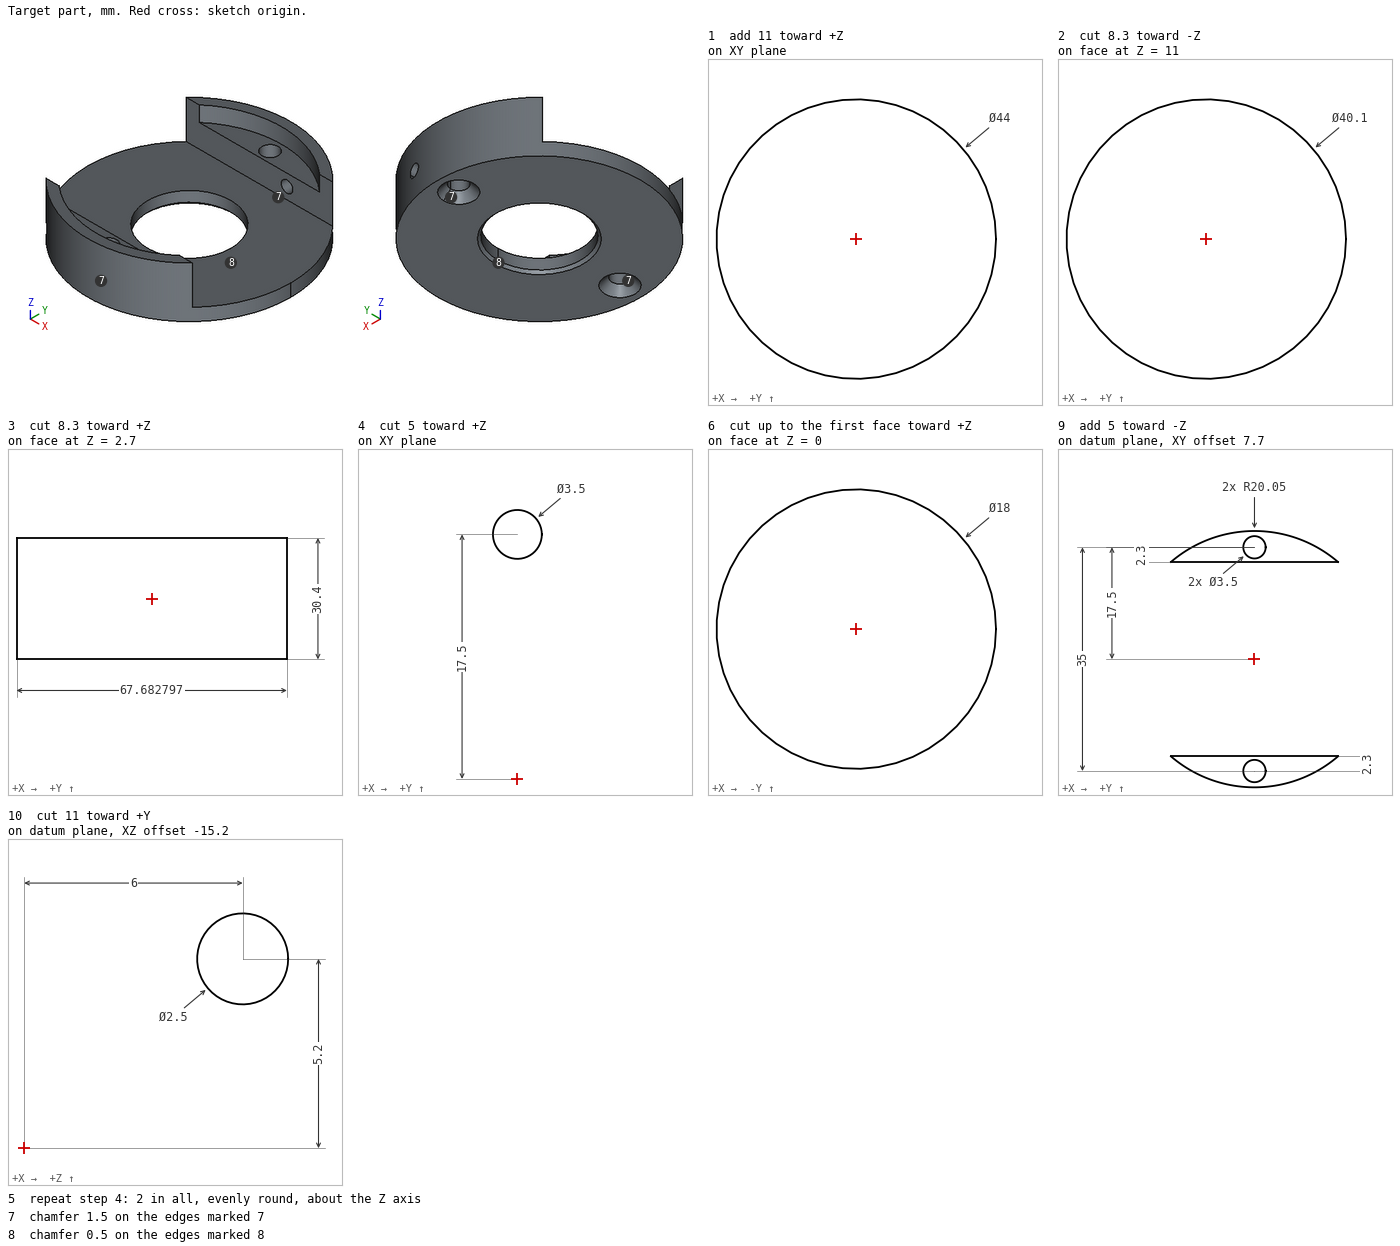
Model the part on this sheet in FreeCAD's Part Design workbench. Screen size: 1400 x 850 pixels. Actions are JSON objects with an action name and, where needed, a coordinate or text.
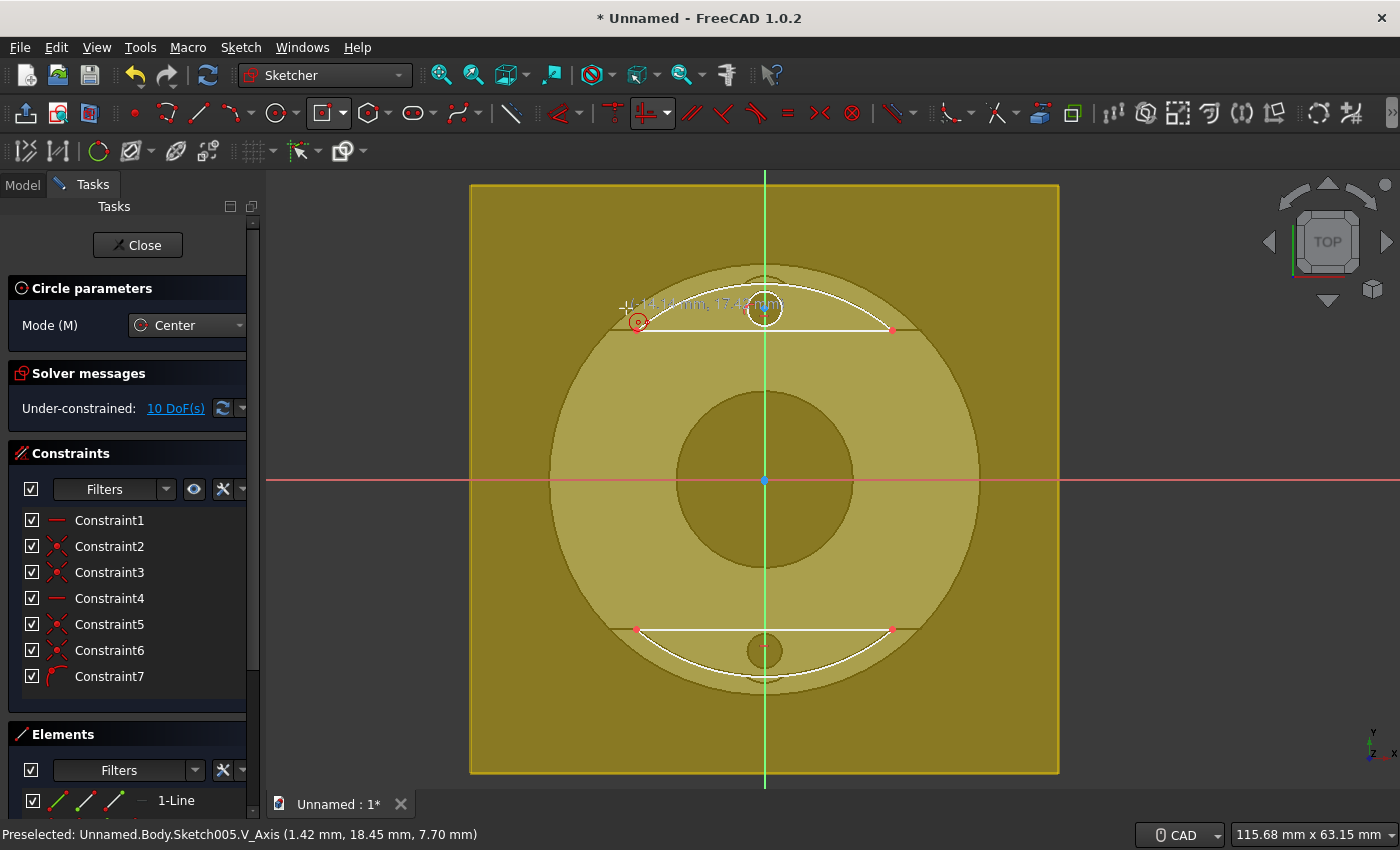
{"action": "scroll", "coordinate": [765, 651], "scroll_direction": "up", "scroll_amount": 2}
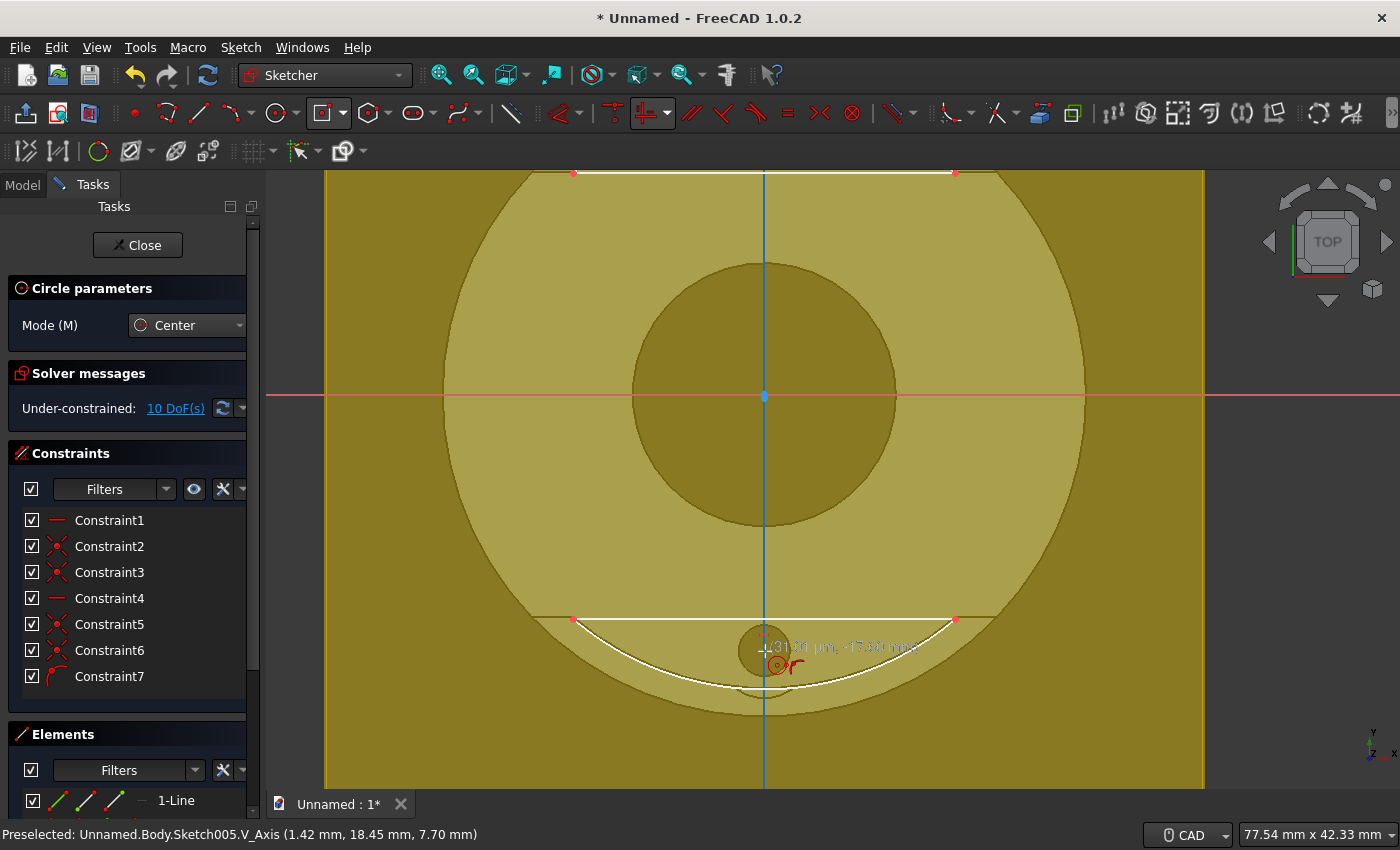
{"action": "left_click", "coordinate": [764, 651]}
{"action": "left_click", "coordinate": [782, 633]}
{"action": "key", "text": "Escape"}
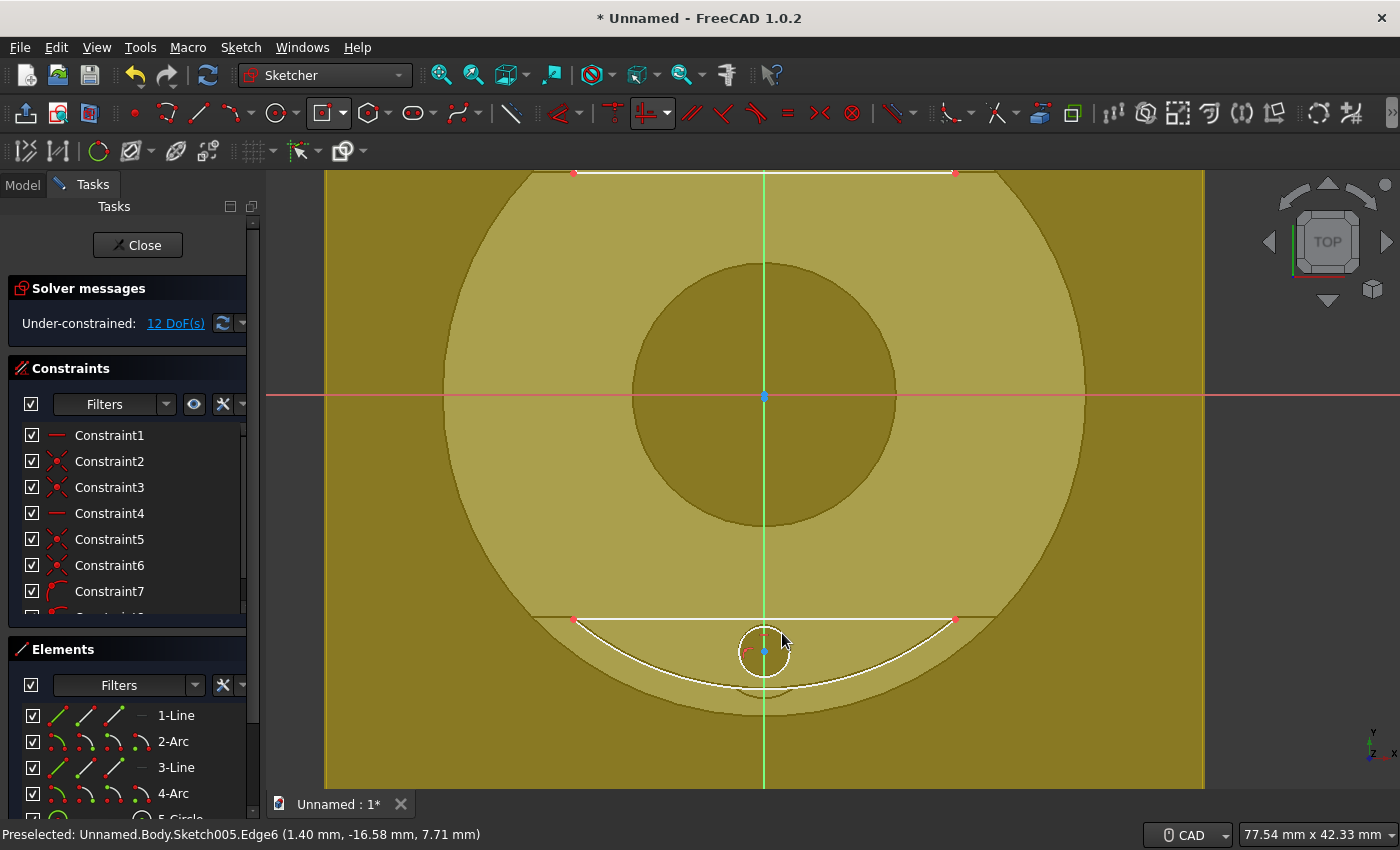
{"action": "scroll", "coordinate": [765, 652], "scroll_direction": "down", "scroll_amount": 2}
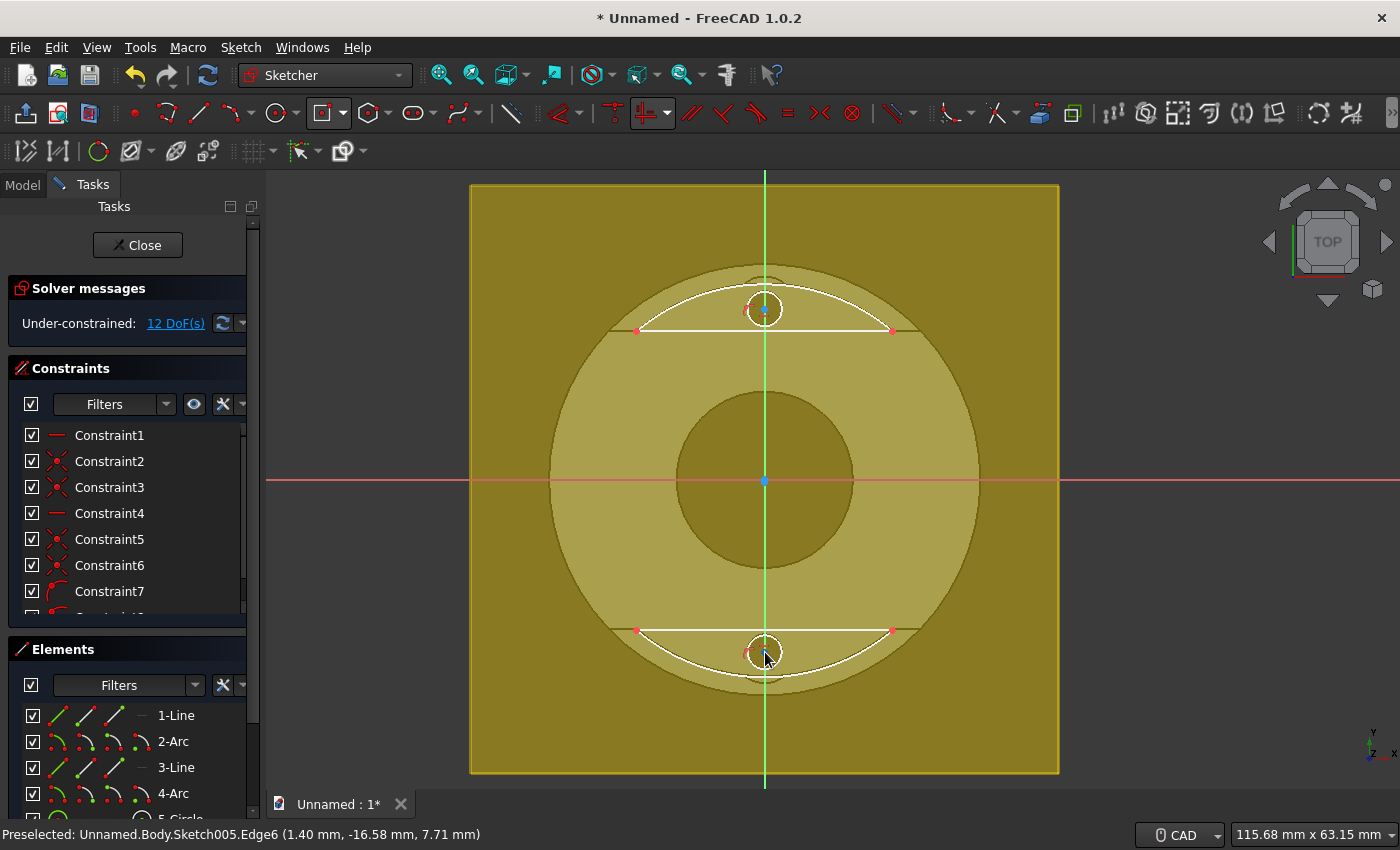
{"action": "left_click", "coordinate": [820, 292]}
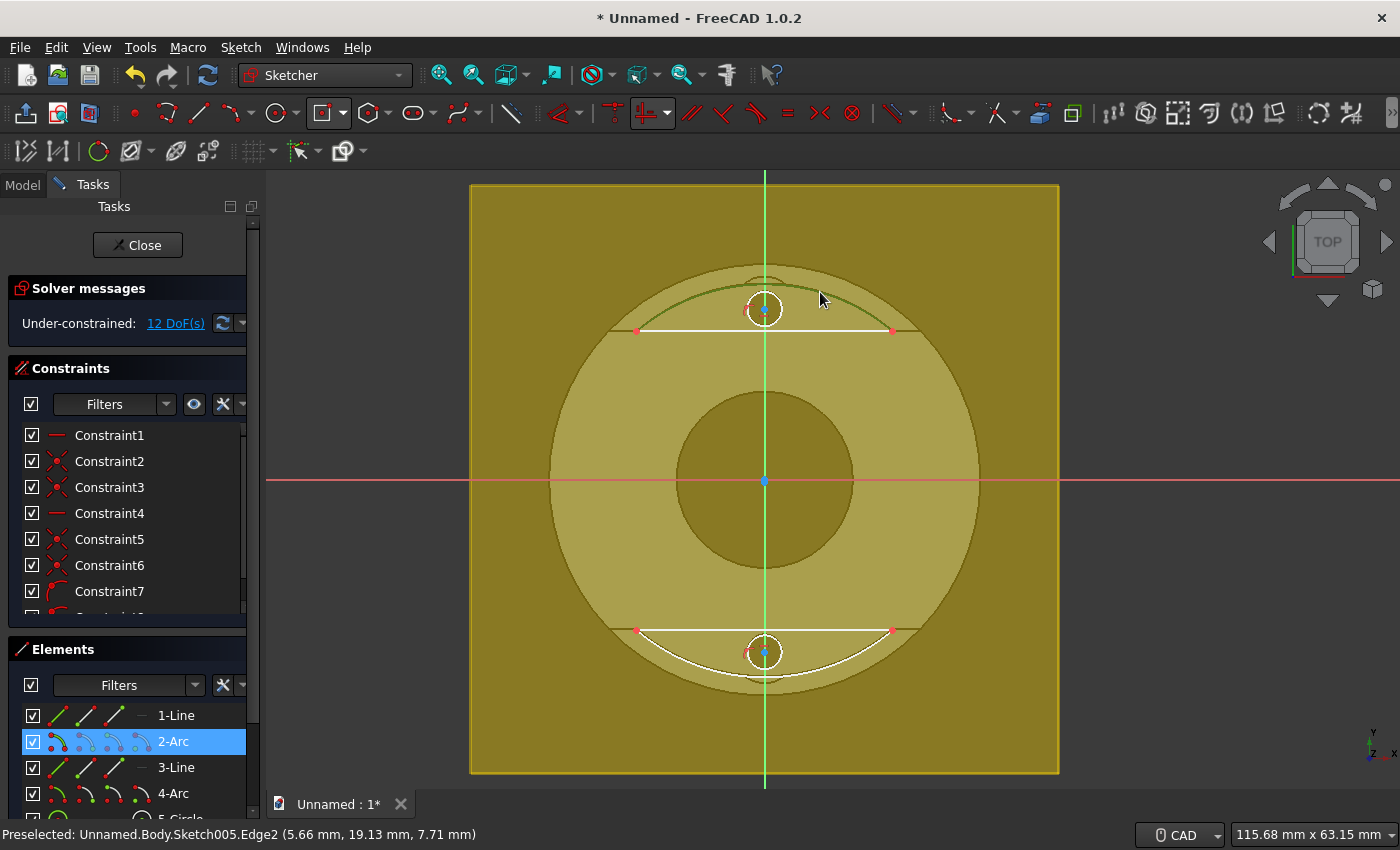
{"action": "left_click", "coordinate": [710, 670]}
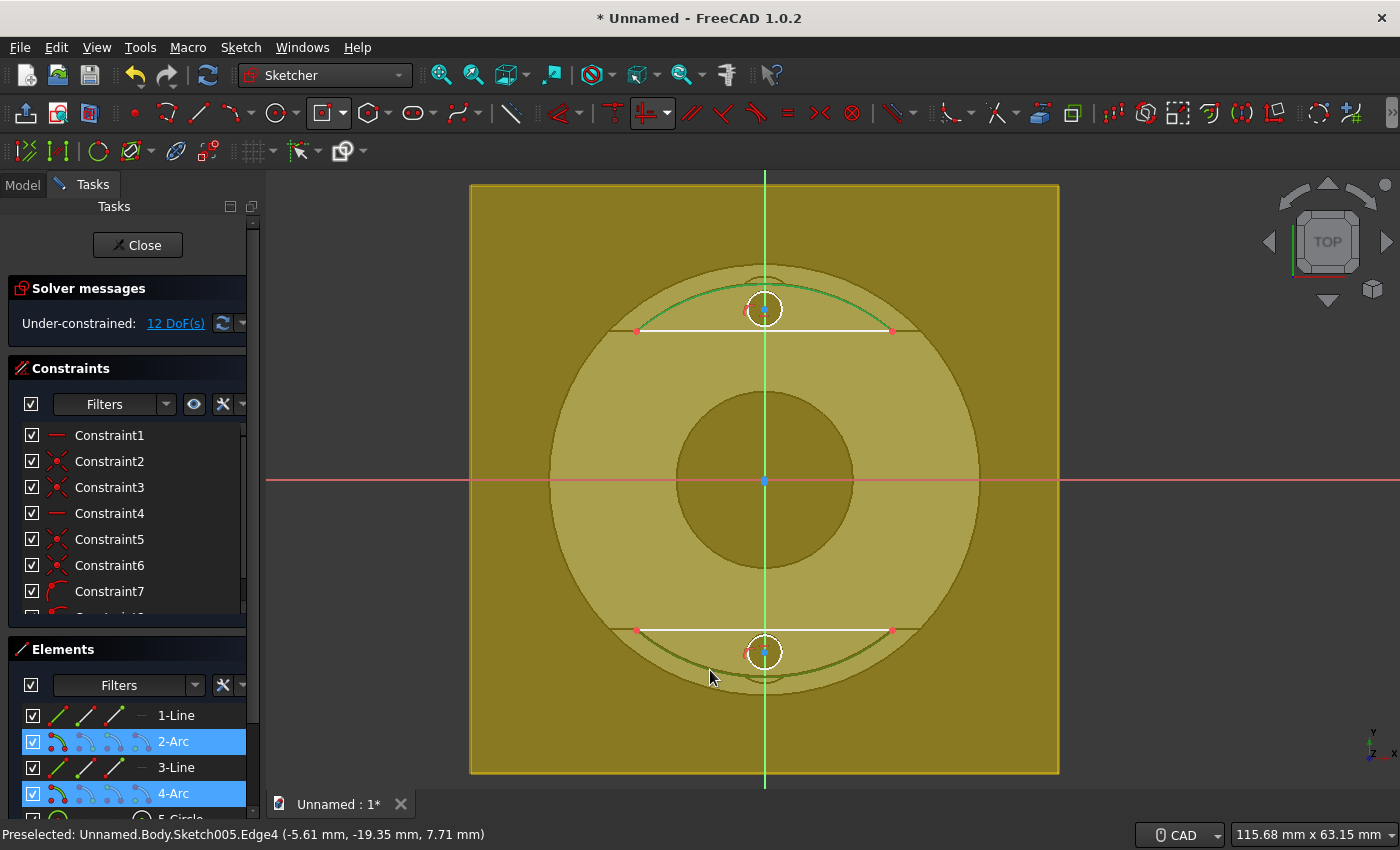
{"action": "key", "text": "c"}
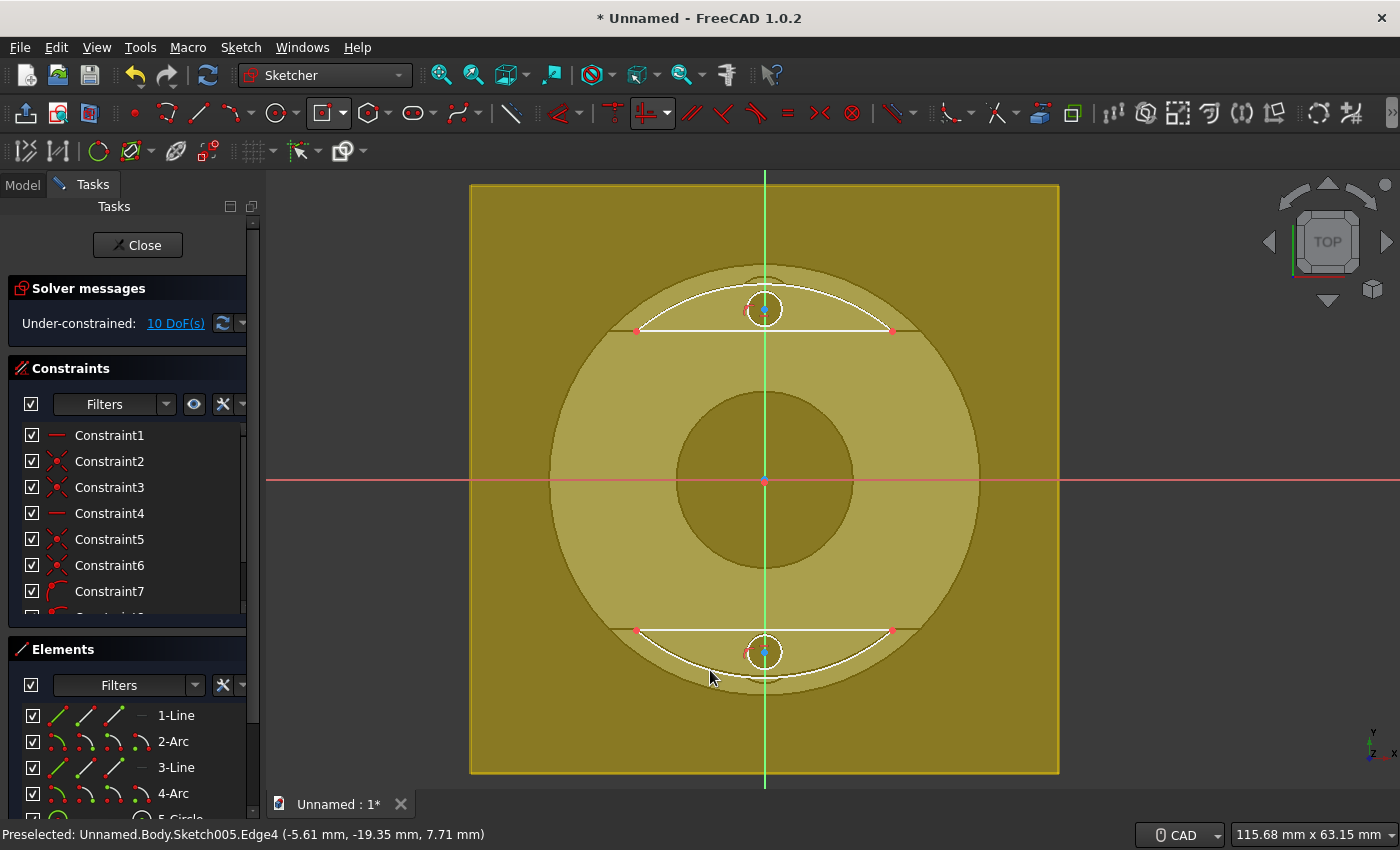
{"action": "scroll", "coordinate": [765, 481], "scroll_direction": "up", "scroll_amount": 5}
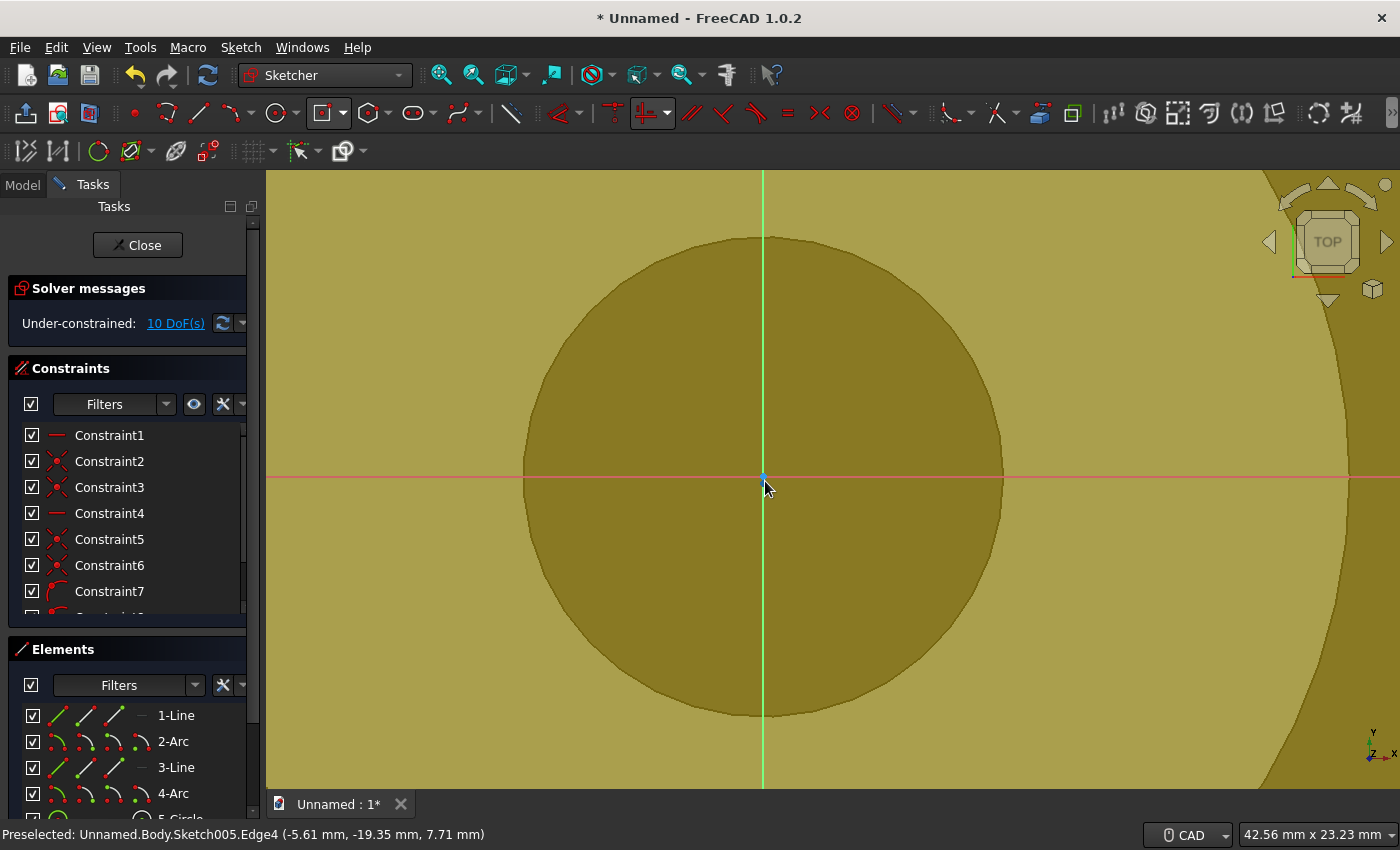
{"action": "left_click_drag", "start_coordinate": [753, 467], "coordinate": [773, 493]}